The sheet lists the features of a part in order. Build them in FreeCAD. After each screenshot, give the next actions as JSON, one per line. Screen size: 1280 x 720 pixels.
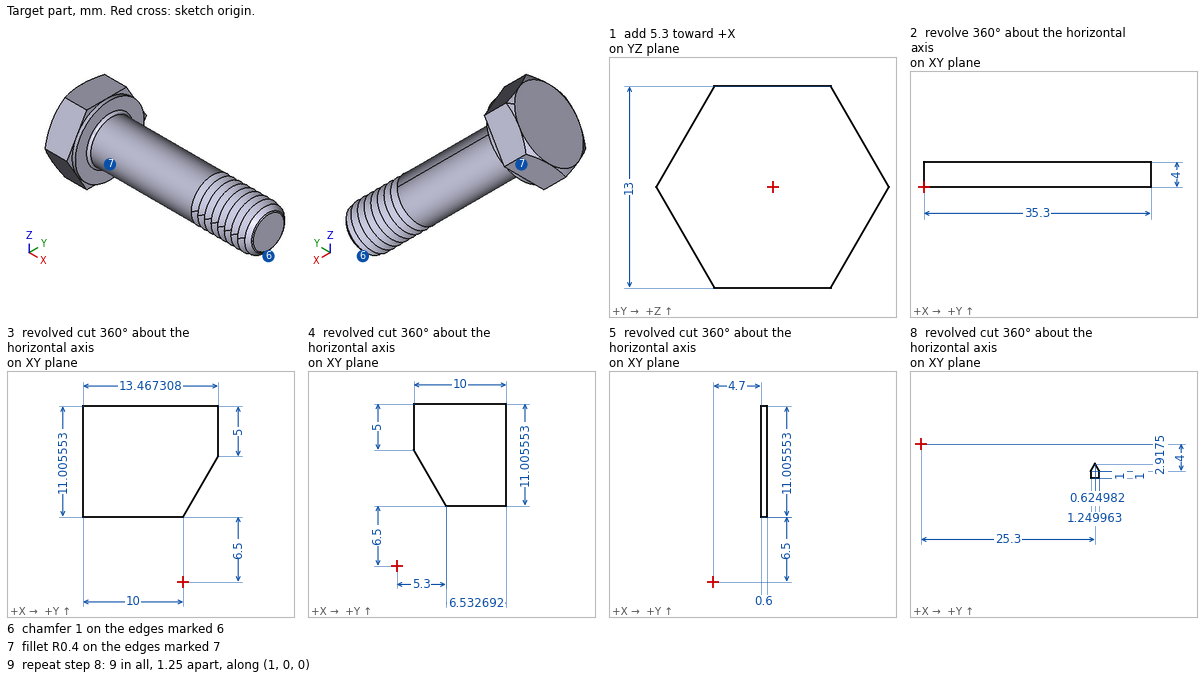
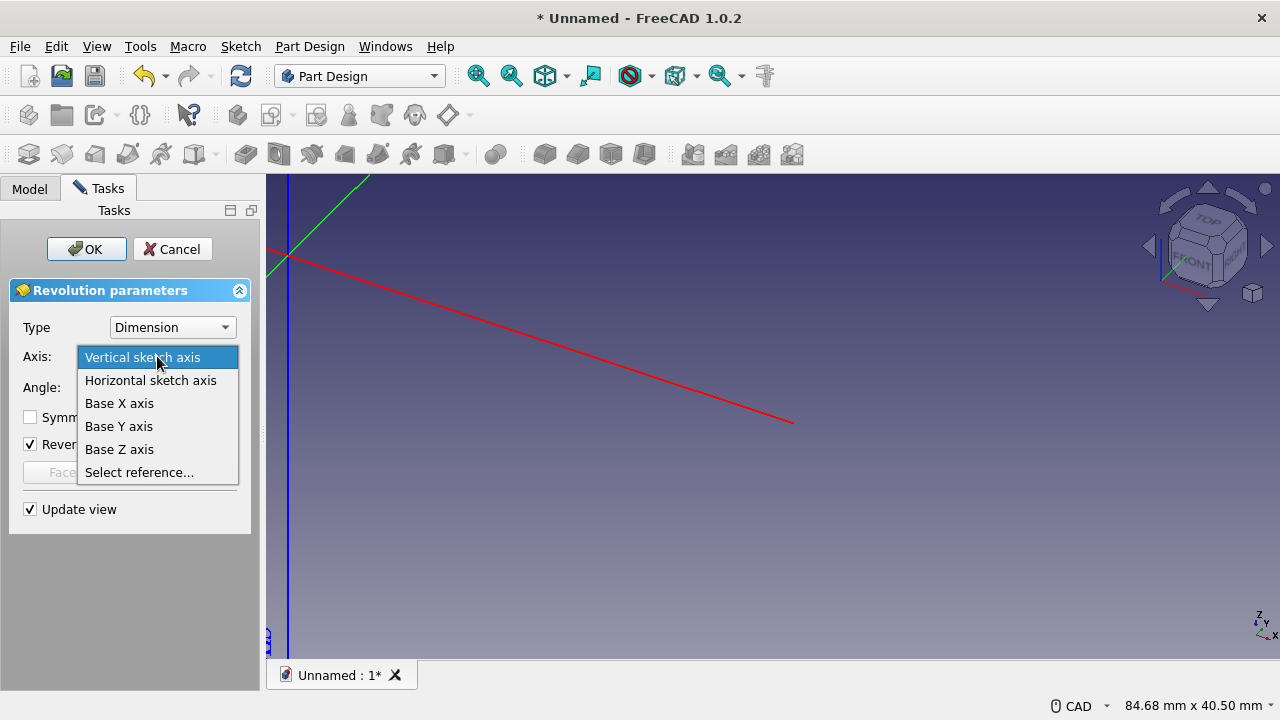
{"action": "left_click", "coordinate": [156, 380]}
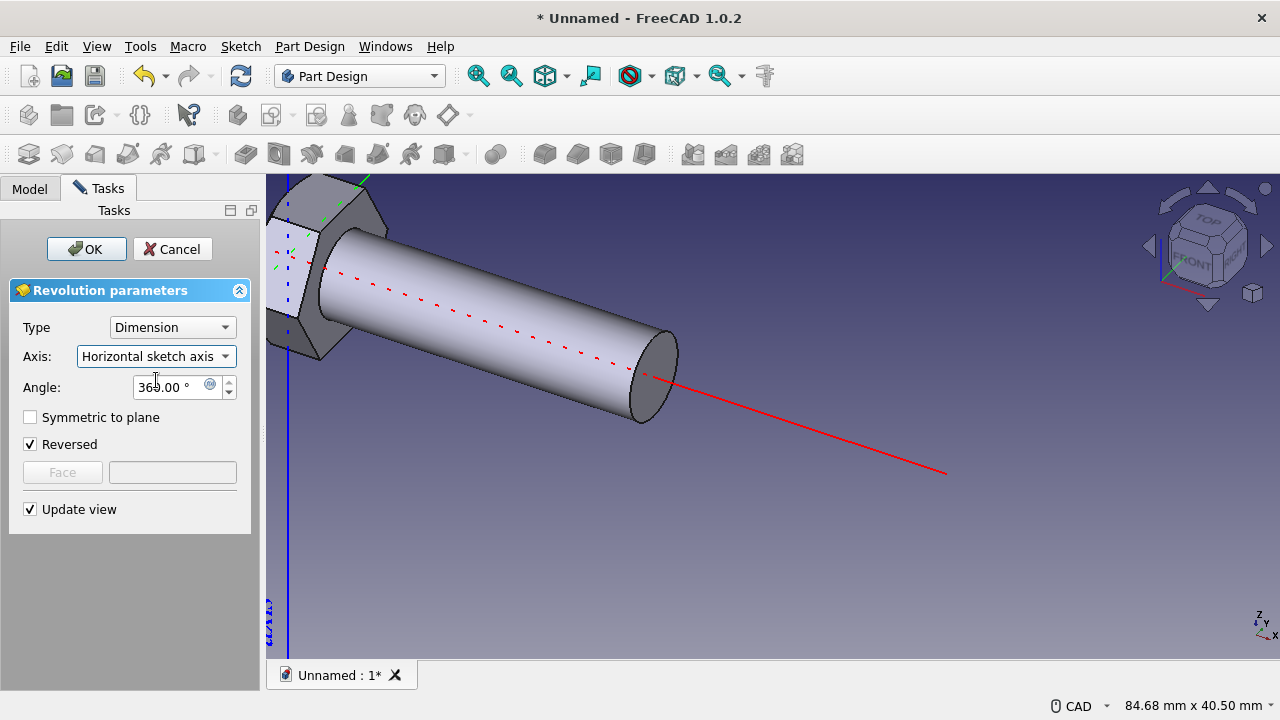
{"action": "left_click", "coordinate": [87, 249]}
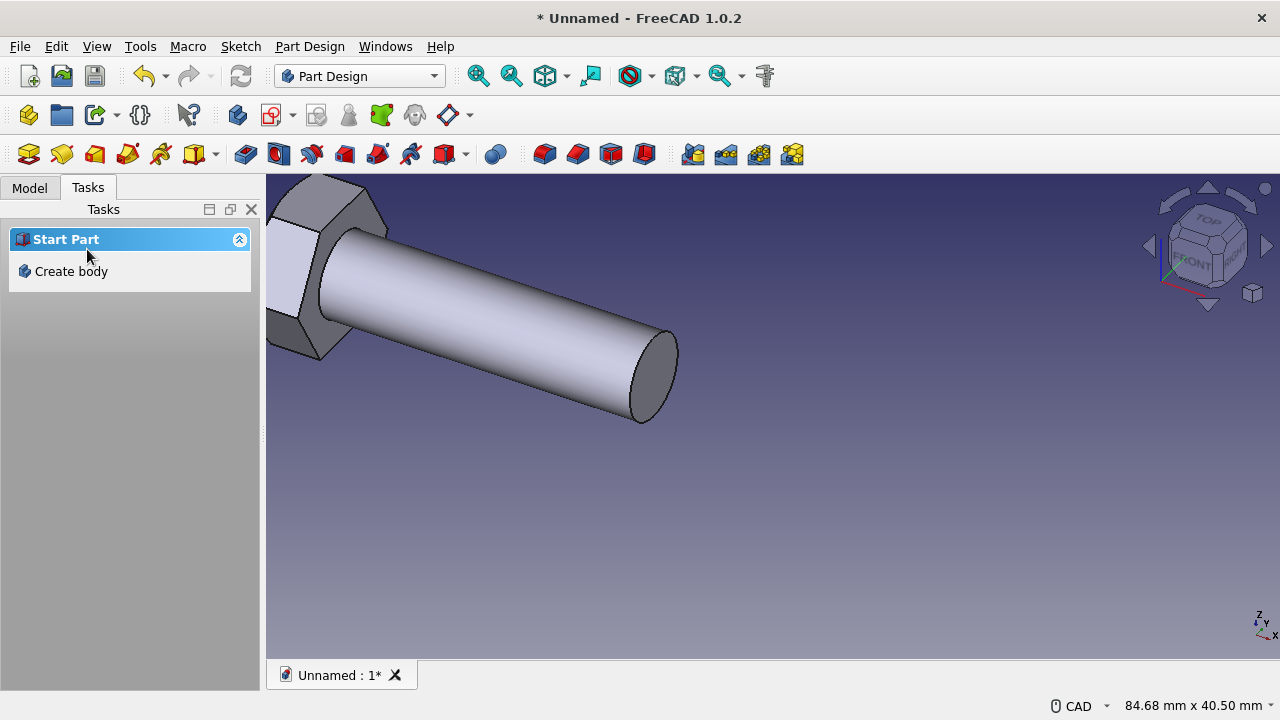
{"action": "left_click", "coordinate": [479, 76]}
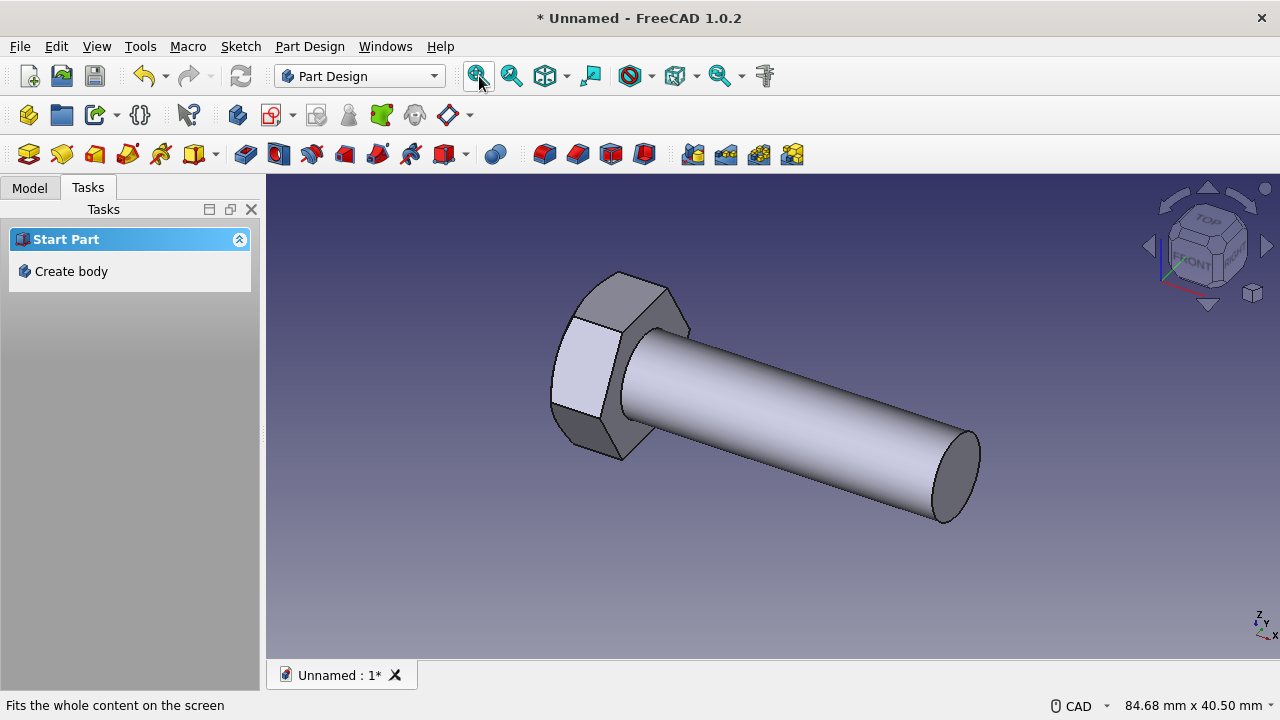
{"action": "left_click", "coordinate": [270, 116]}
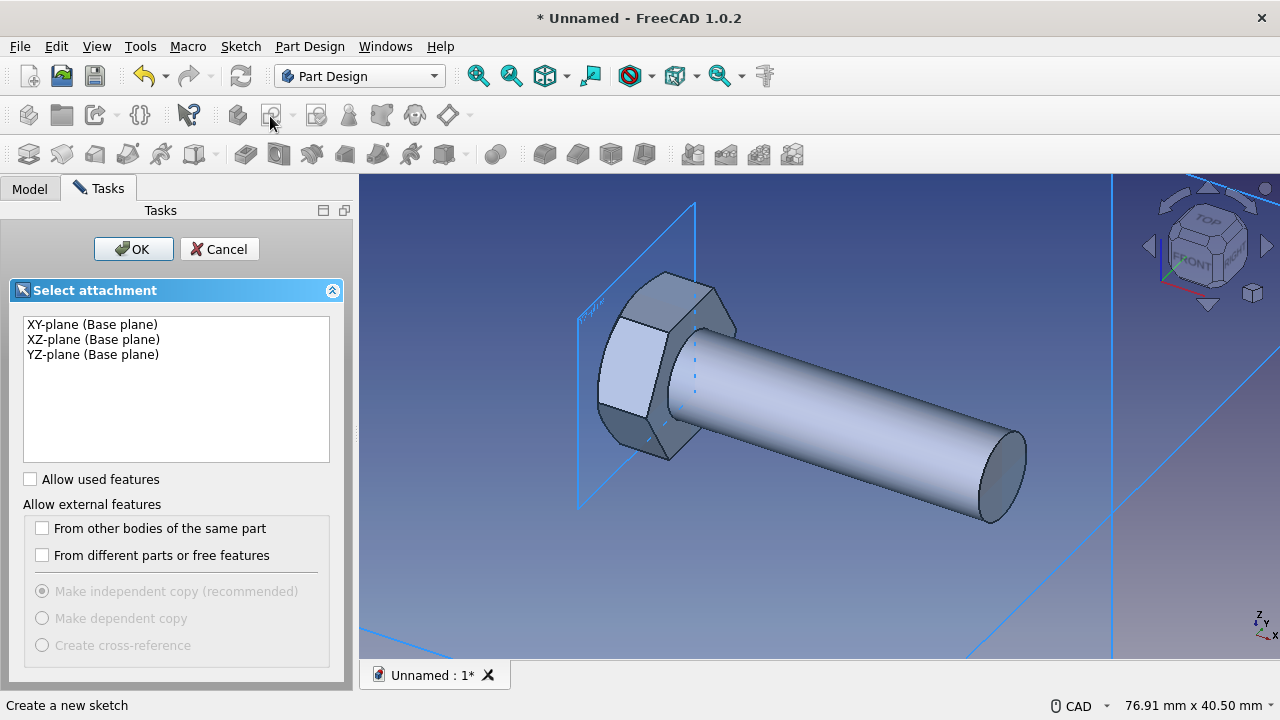
{"action": "left_click", "coordinate": [84, 324]}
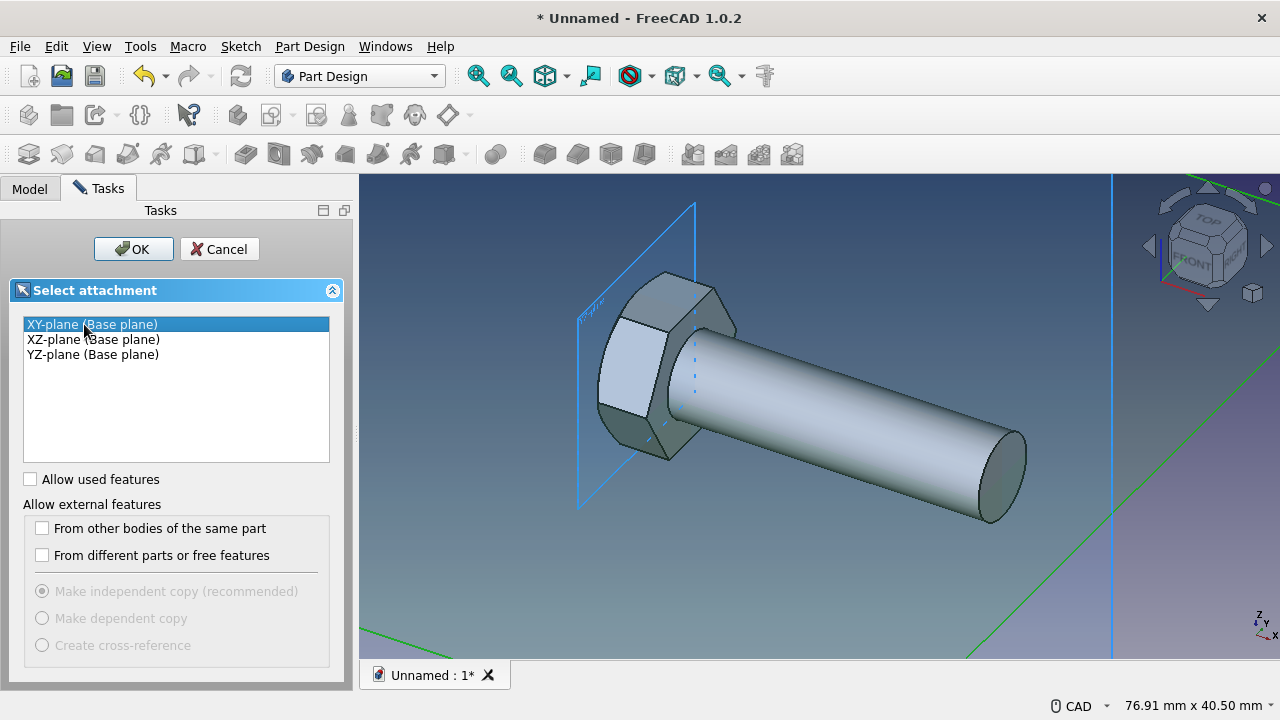
{"action": "left_click", "coordinate": [134, 249]}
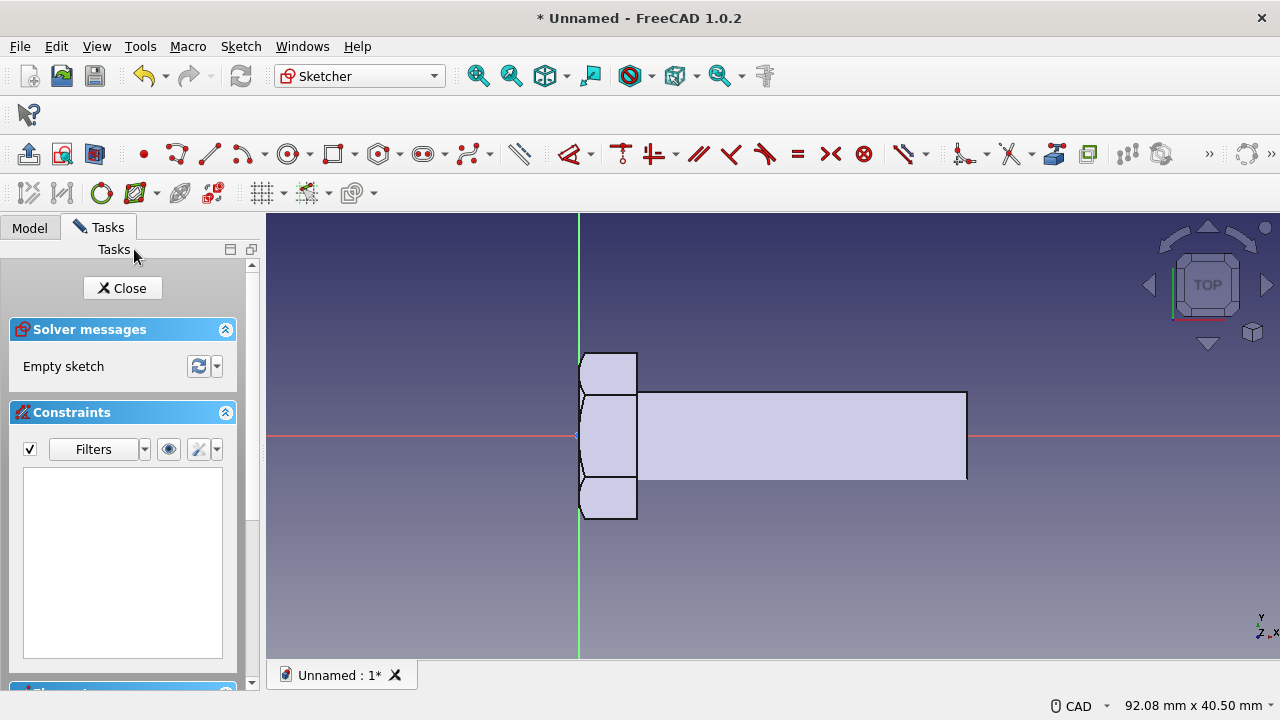
{"action": "left_click", "coordinate": [95, 154]}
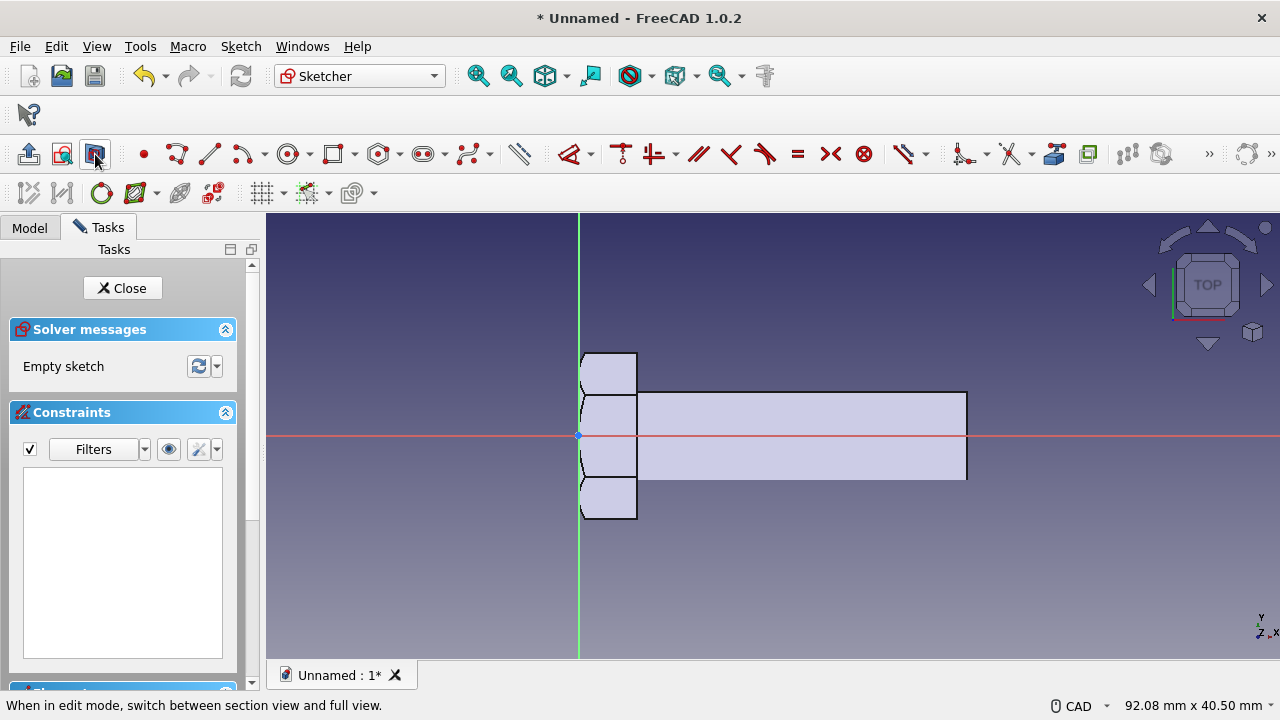
{"action": "scroll", "coordinate": [979, 631], "scroll_direction": "down", "scroll_amount": 1}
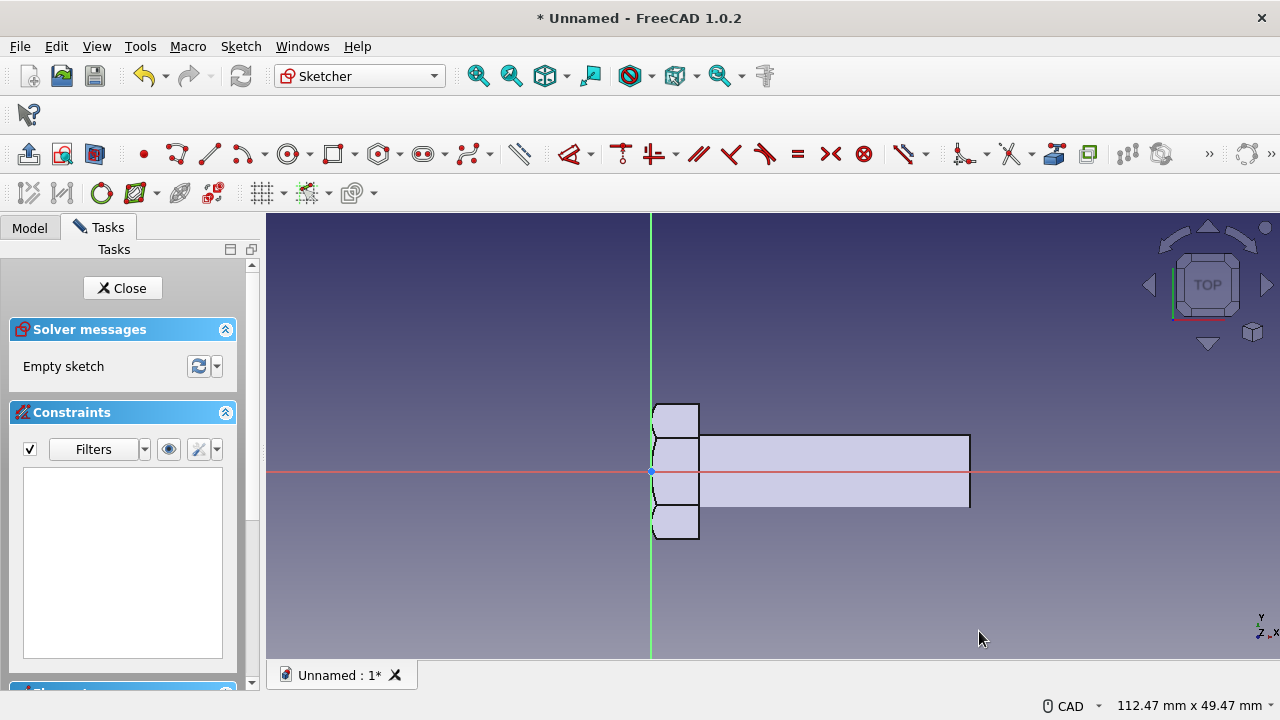
{"action": "scroll", "coordinate": [705, 340], "scroll_direction": "up", "scroll_amount": 3}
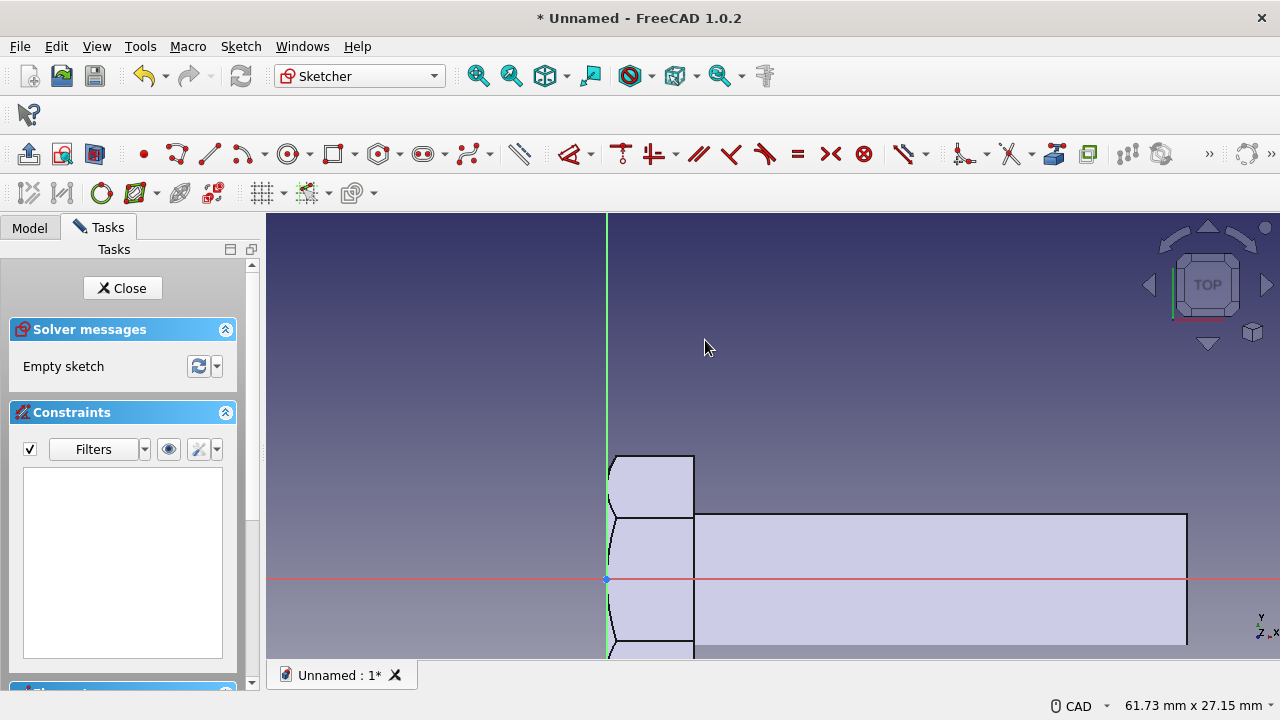
{"action": "left_click", "coordinate": [177, 154]}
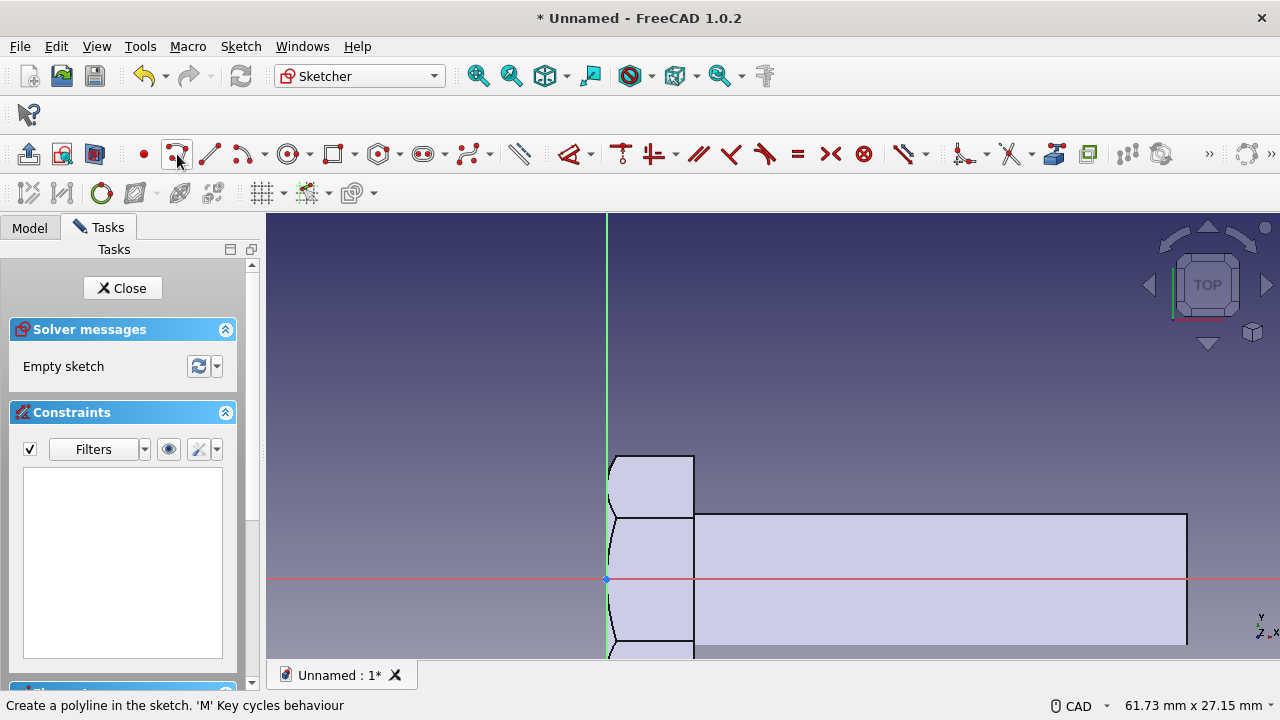
{"action": "left_click", "coordinate": [694, 473]}
{"action": "left_click", "coordinate": [801, 473]}
{"action": "left_click", "coordinate": [801, 292]}
{"action": "left_click", "coordinate": [637, 292]}
{"action": "left_click", "coordinate": [637, 374]}
{"action": "left_click", "coordinate": [694, 474]}
{"action": "key", "text": "Escape"}
{"action": "key", "text": "Escape"}